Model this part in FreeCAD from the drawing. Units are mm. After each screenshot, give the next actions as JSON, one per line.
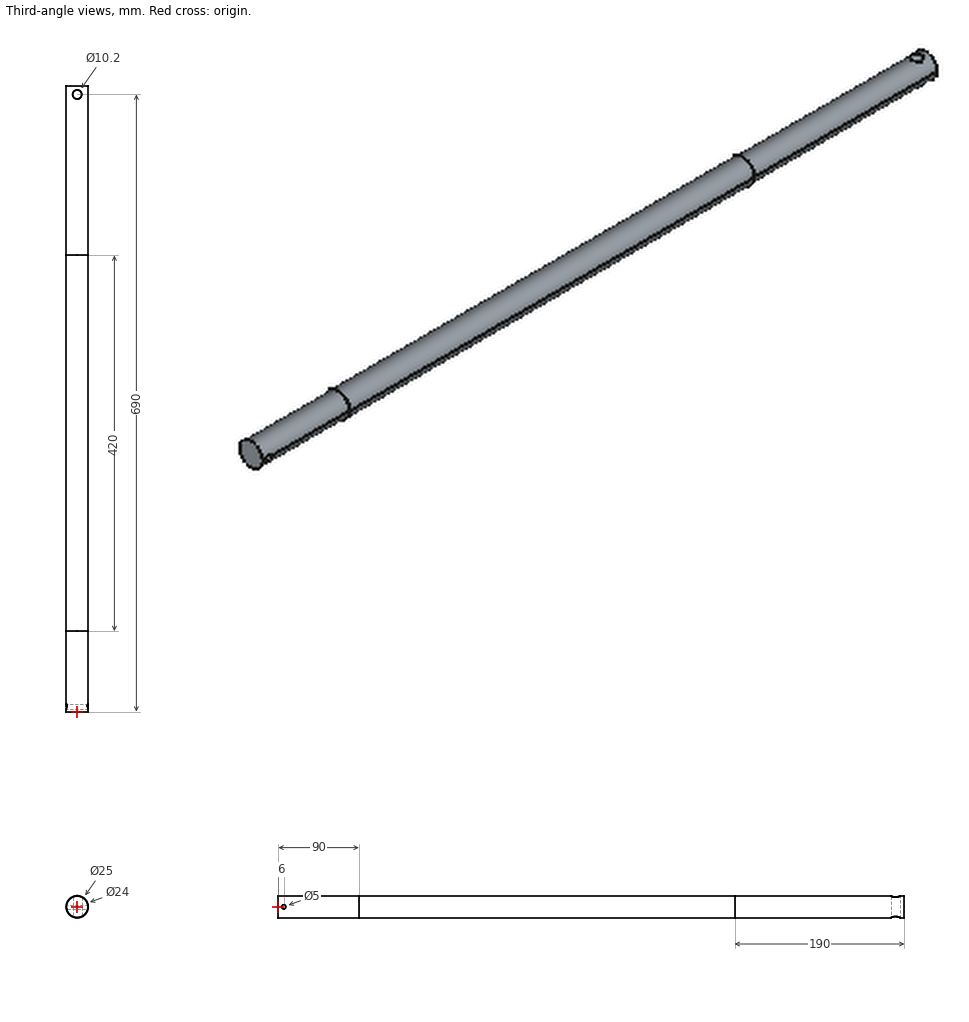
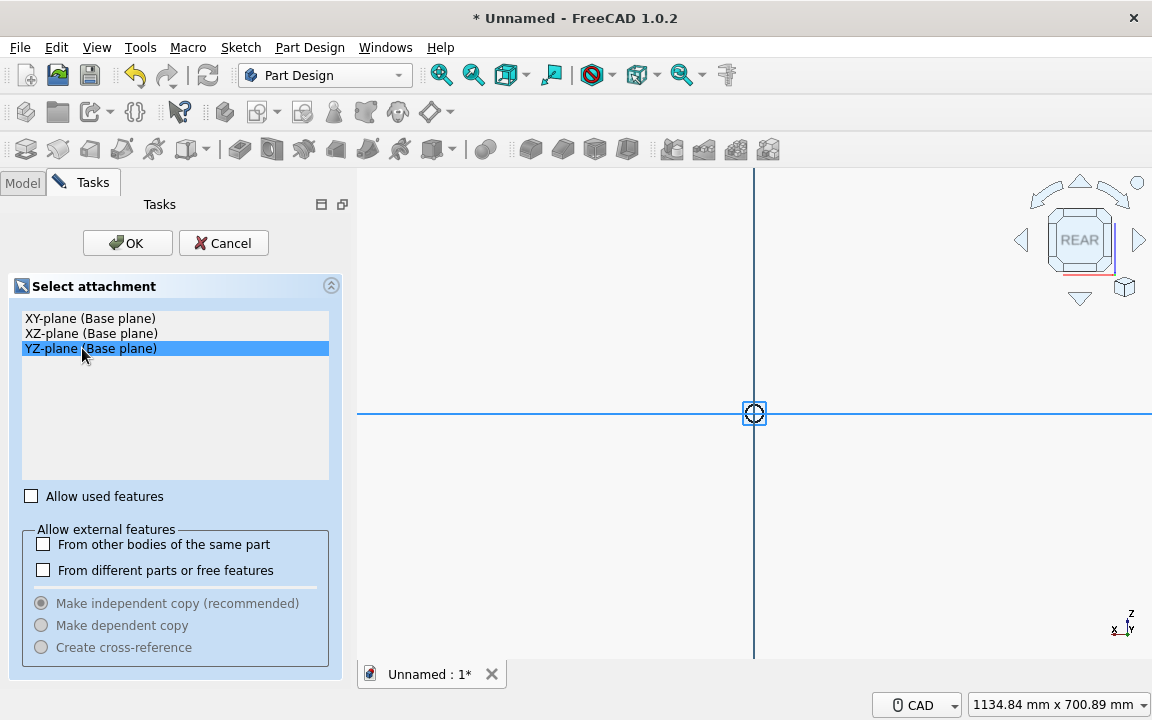
{"action": "left_click", "coordinate": [128, 243]}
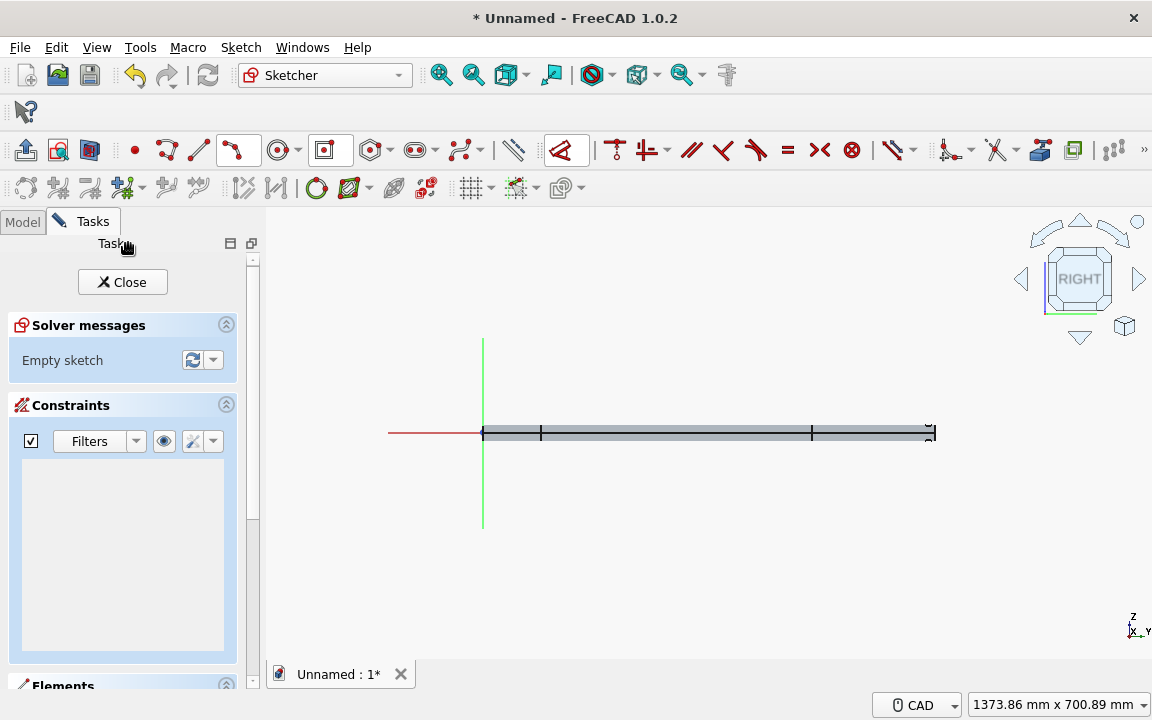
{"action": "left_click", "coordinate": [90, 150]}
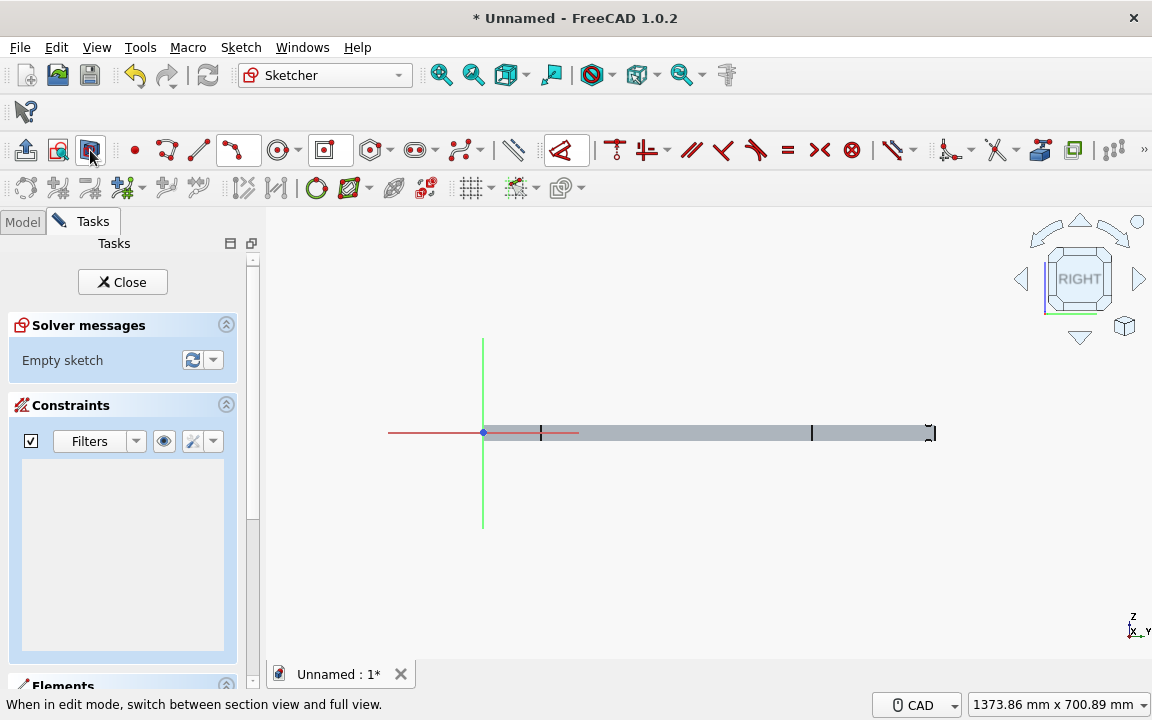
{"action": "scroll", "coordinate": [478, 433], "scroll_direction": "up", "scroll_amount": 15}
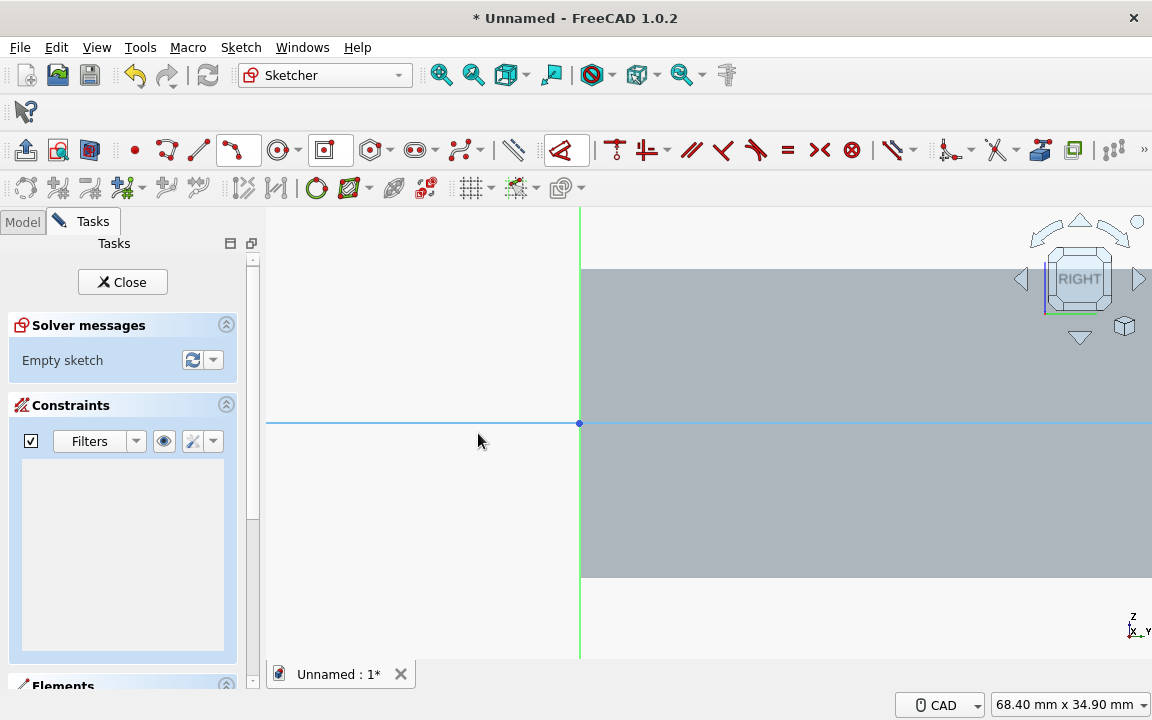
{"action": "scroll", "coordinate": [633, 420], "scroll_direction": "up", "scroll_amount": 7}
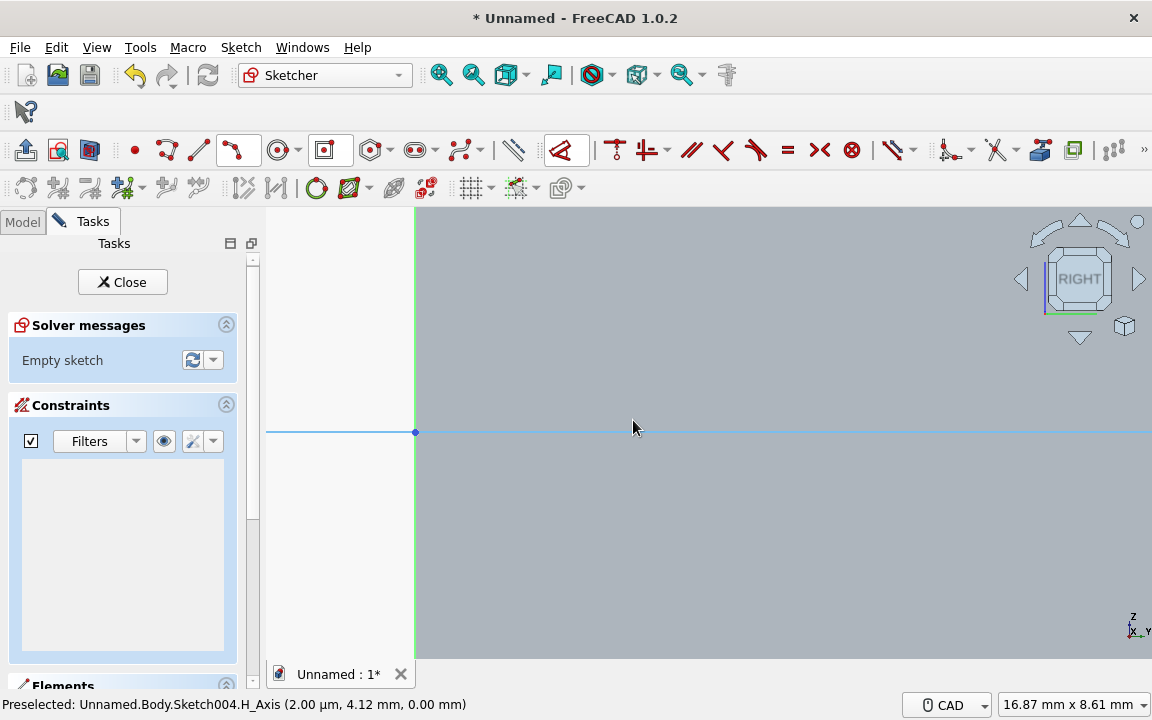
{"action": "key", "text": "g c"}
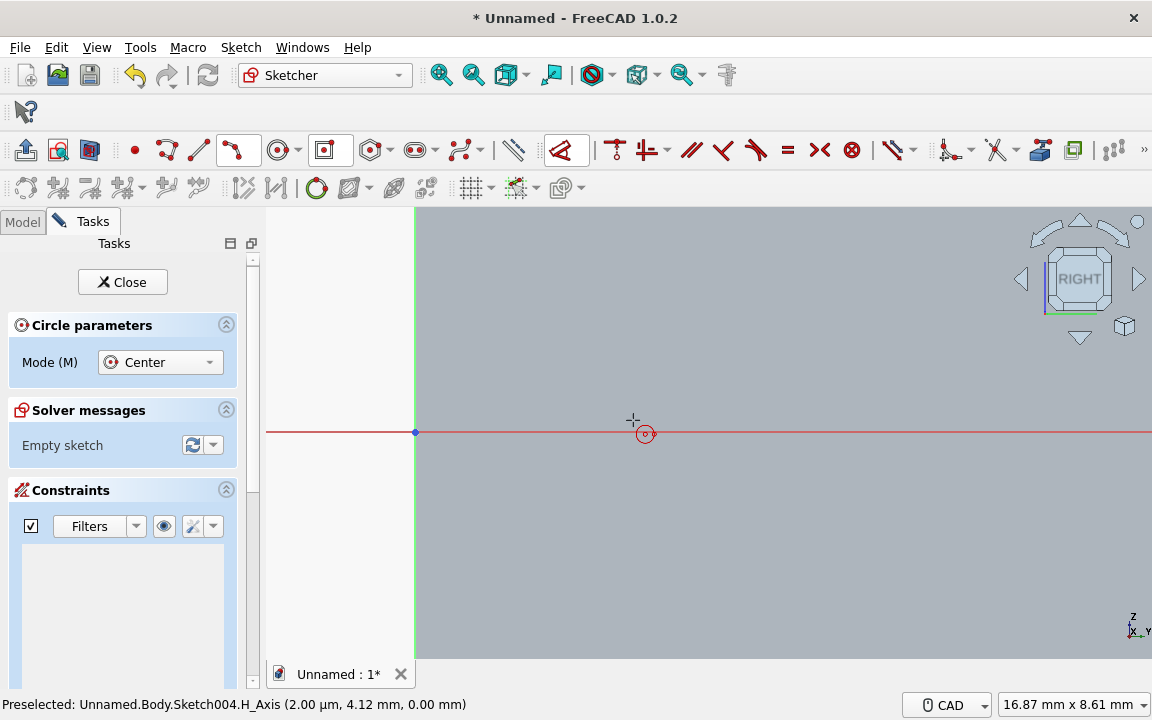
{"action": "left_click", "coordinate": [730, 432]}
{"action": "left_click", "coordinate": [823, 340]}
{"action": "key", "text": "Escape"}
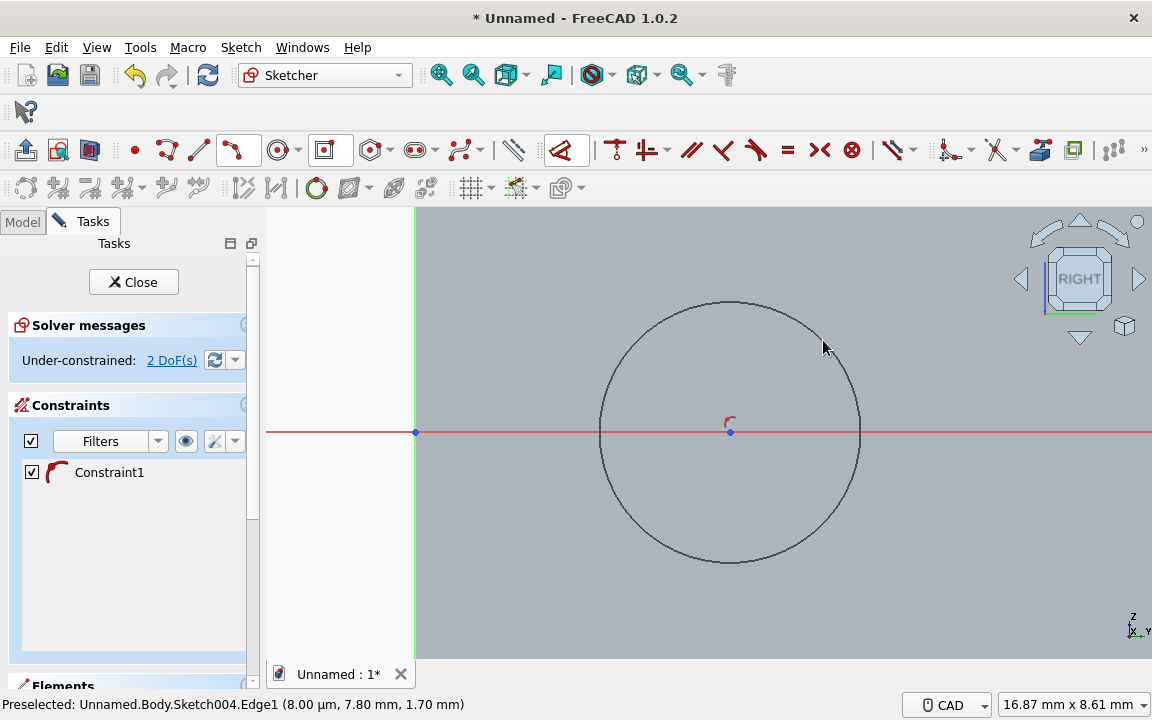
{"action": "left_click", "coordinate": [822, 340]}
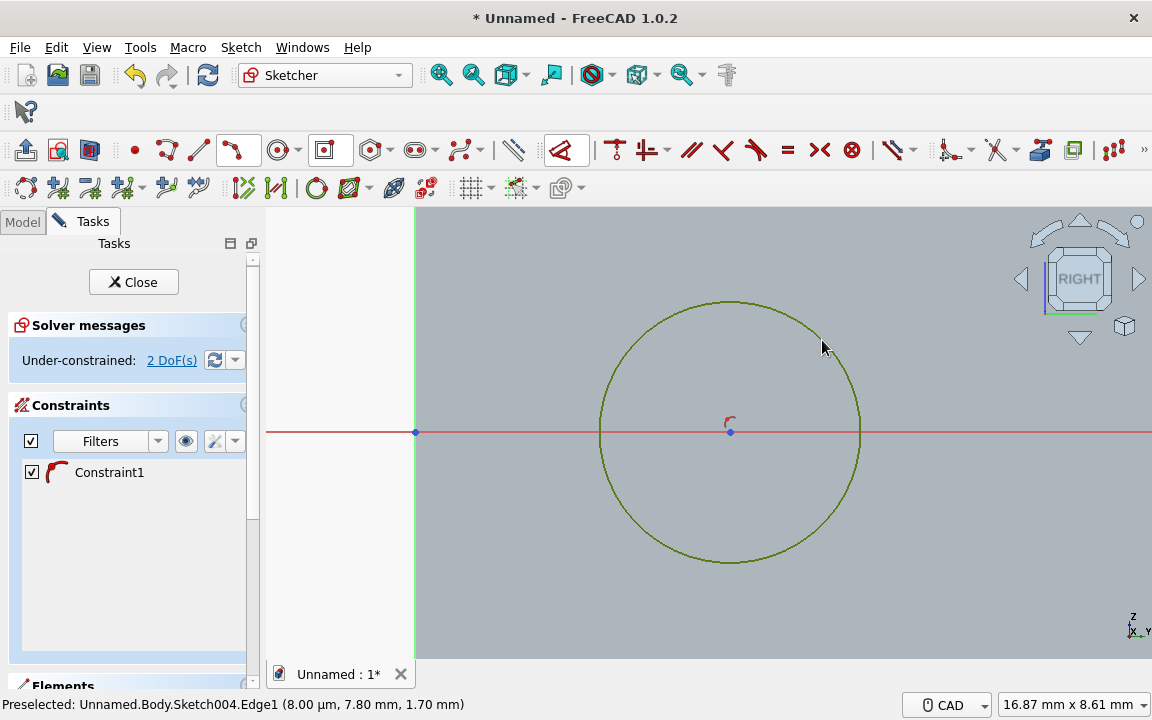
{"action": "left_click", "coordinate": [584, 150]}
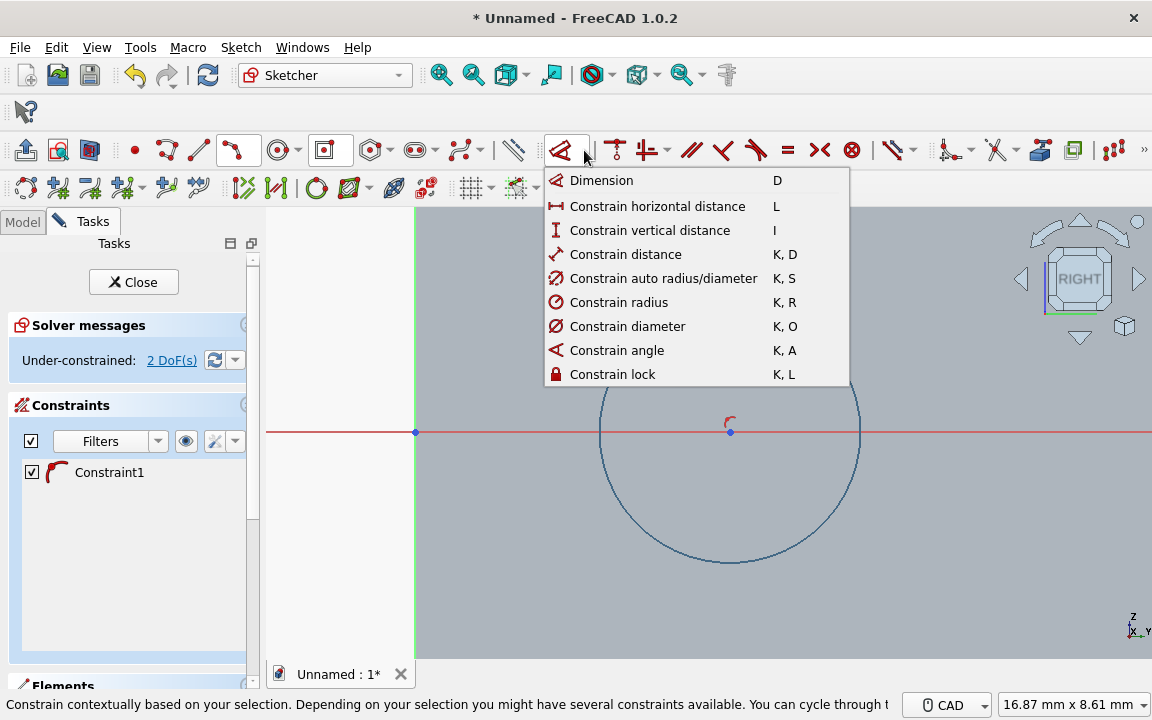
{"action": "left_click", "coordinate": [697, 326]}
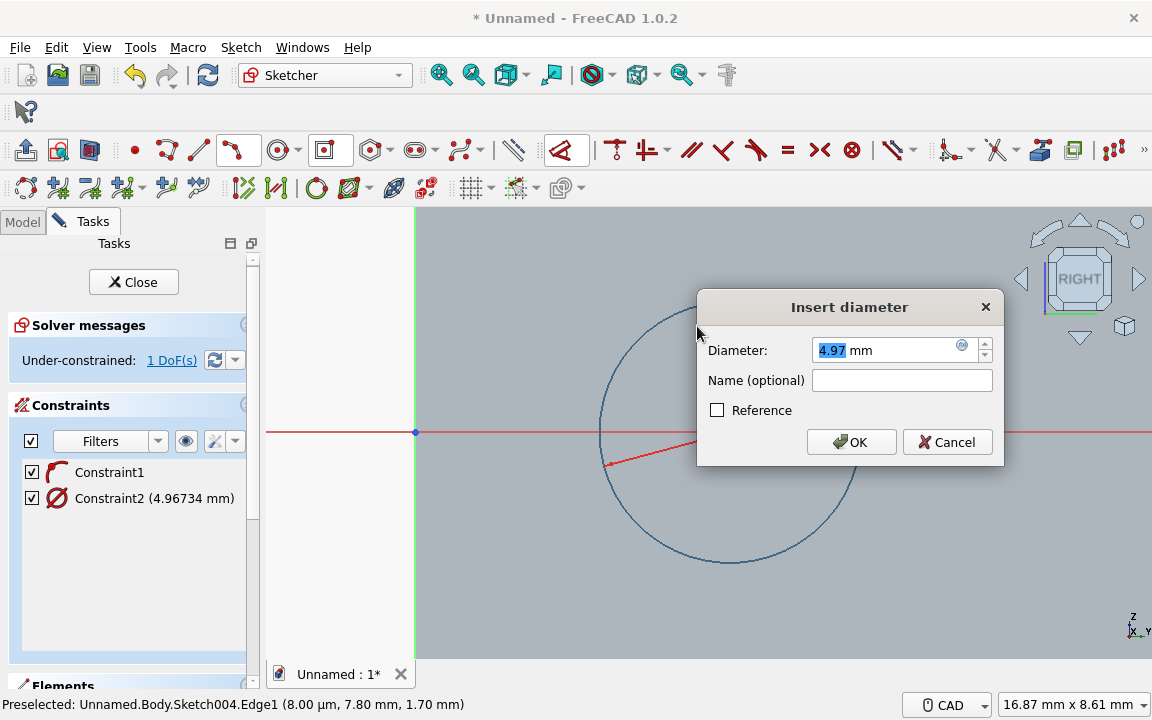
{"action": "type", "text": "5"}
{"action": "key", "text": "Return"}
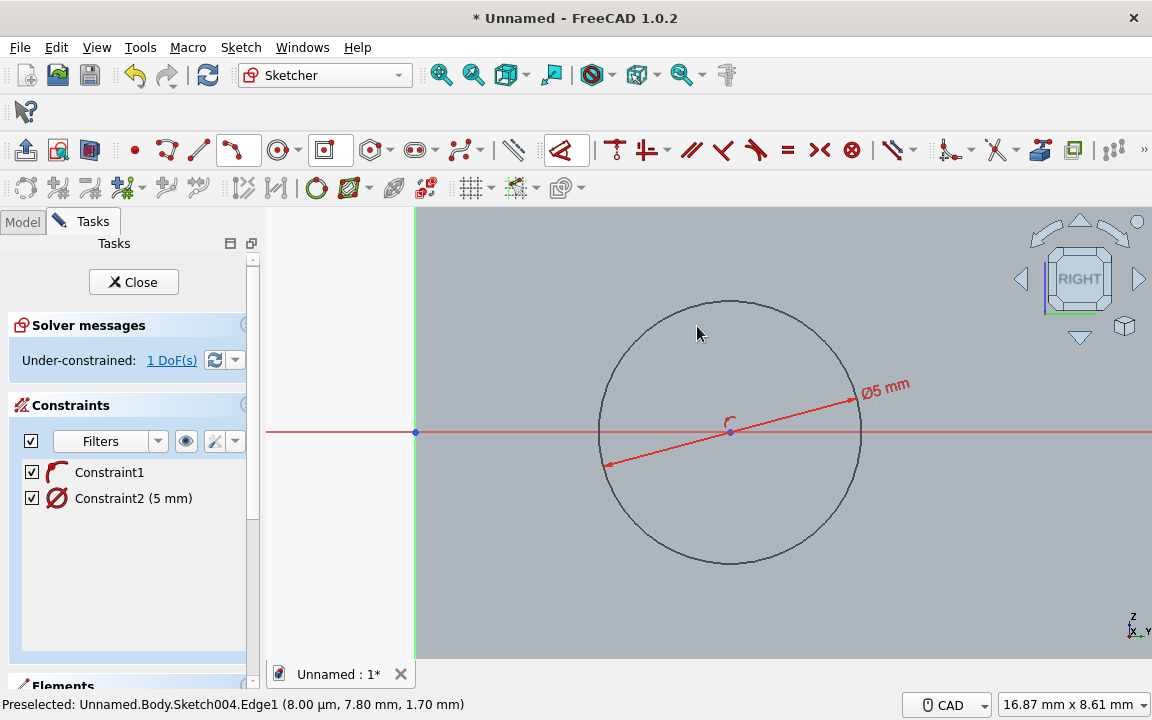
{"action": "left_click", "coordinate": [730, 432]}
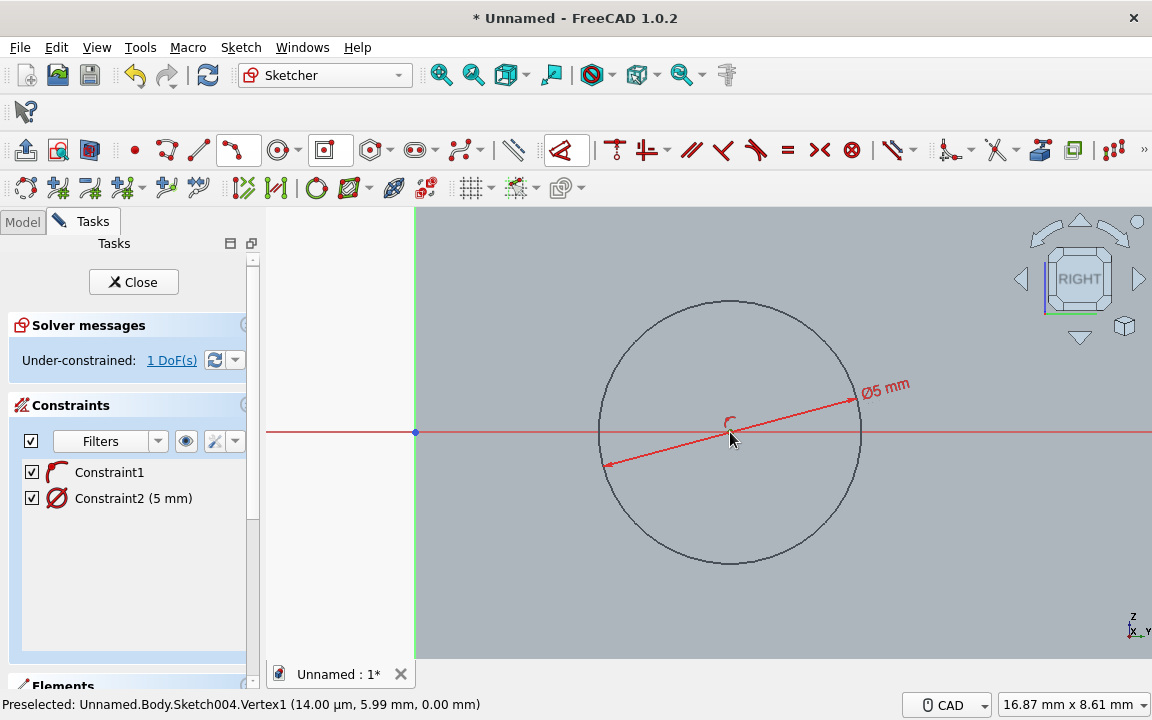
{"action": "left_click", "coordinate": [584, 150]}